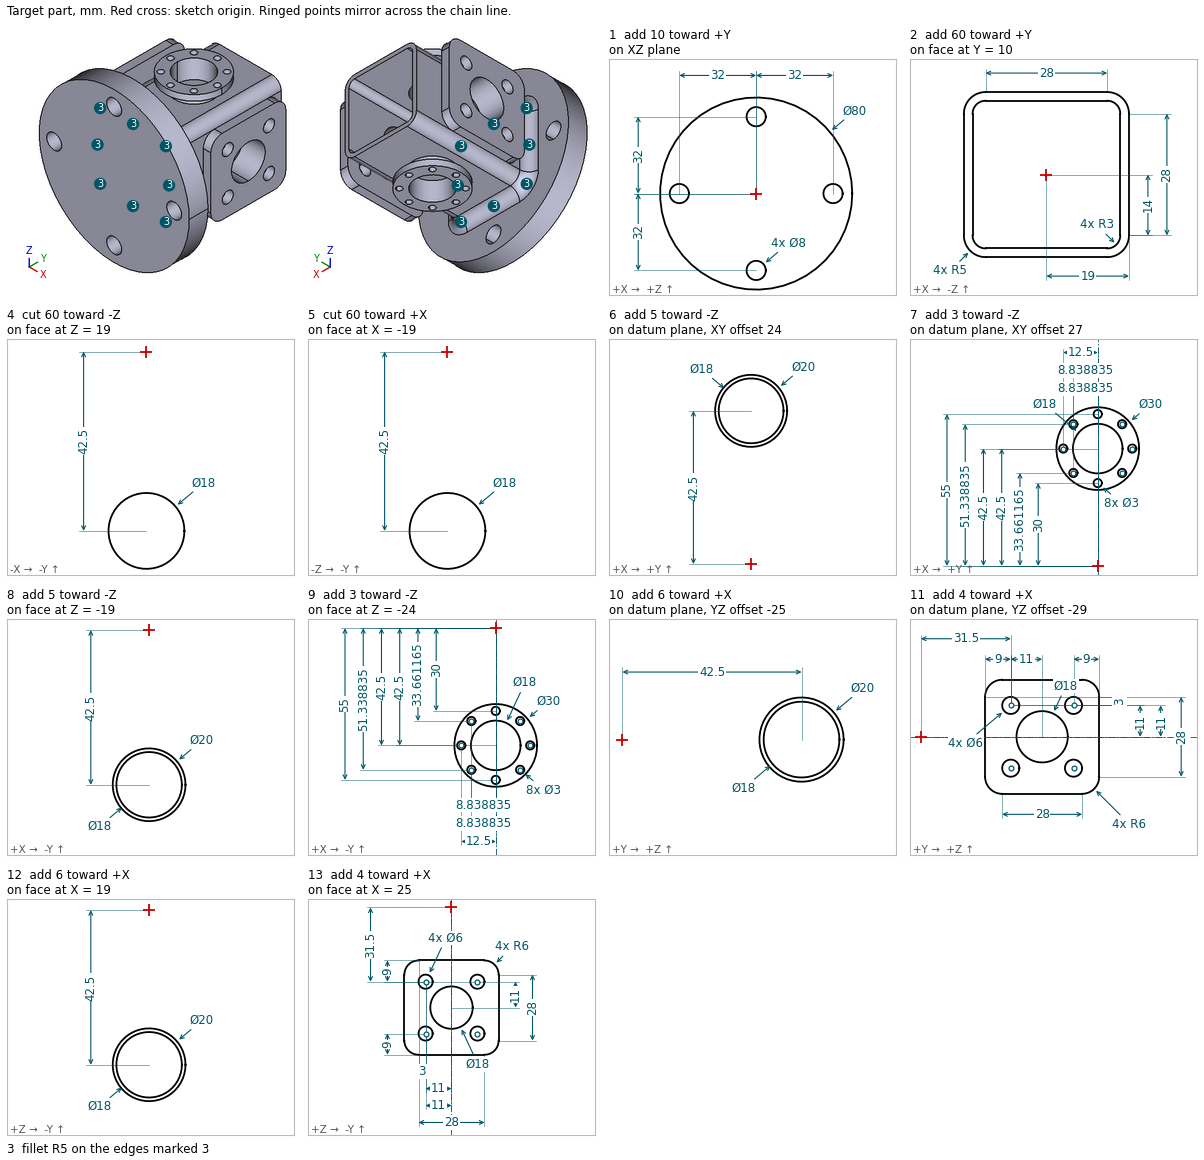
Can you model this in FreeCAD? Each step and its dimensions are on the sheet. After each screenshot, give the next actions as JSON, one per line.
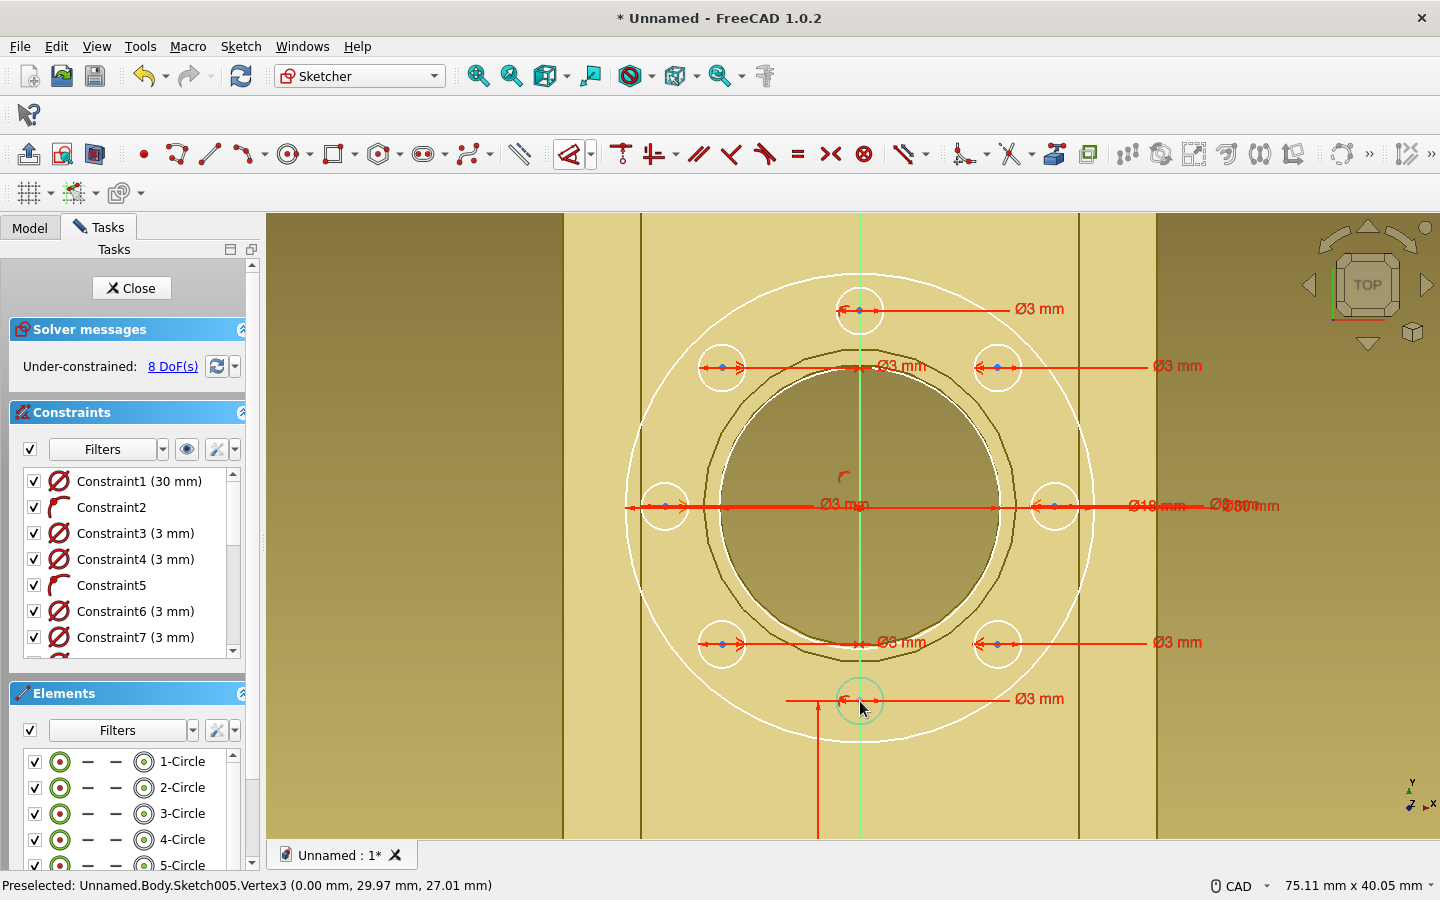
{"action": "left_click", "coordinate": [860, 311]}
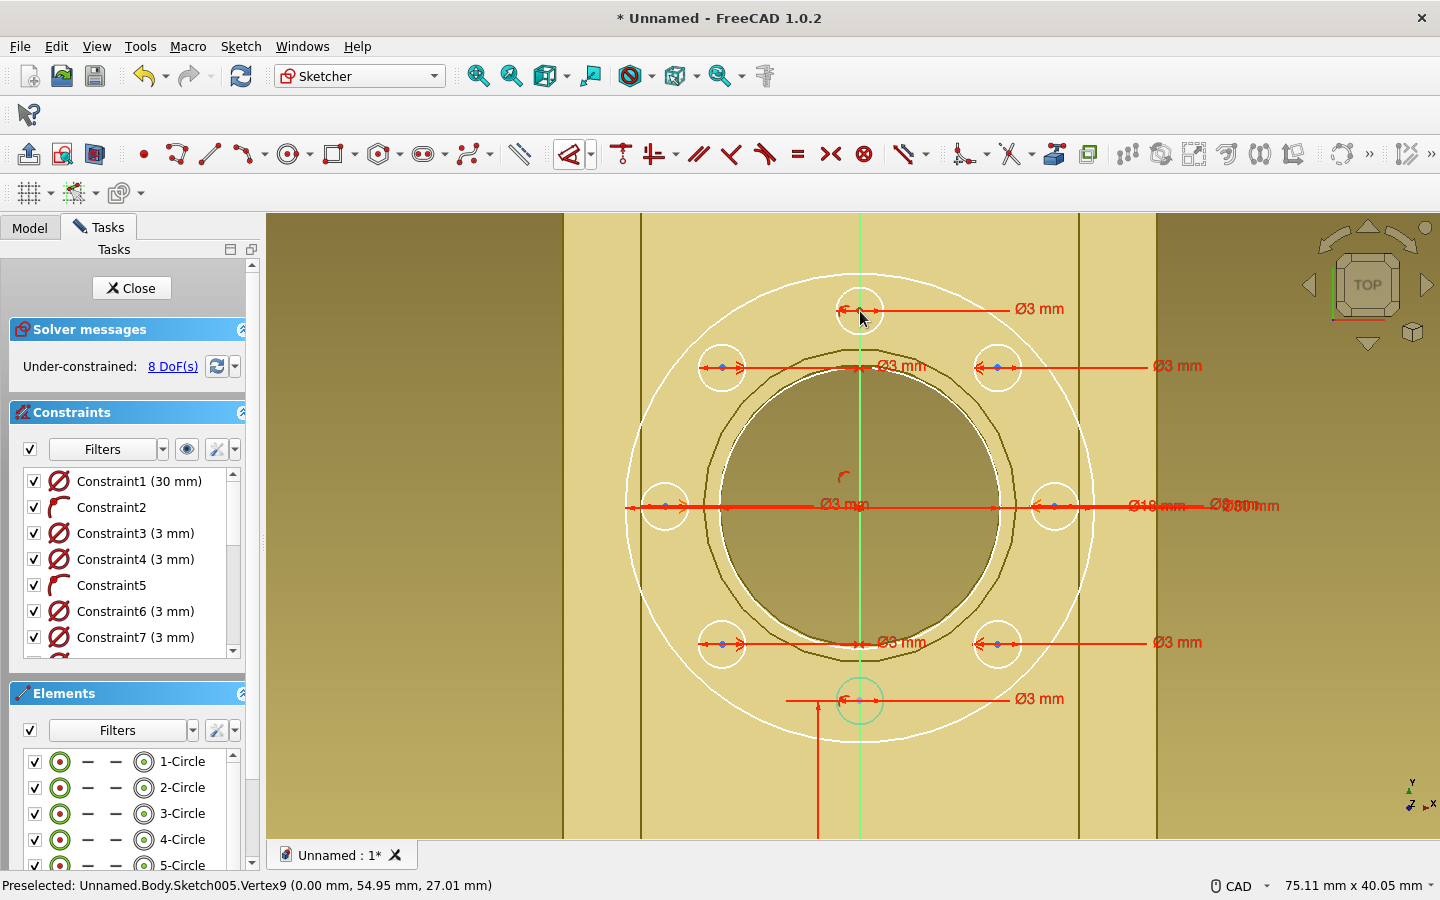
{"action": "key", "text": "i"}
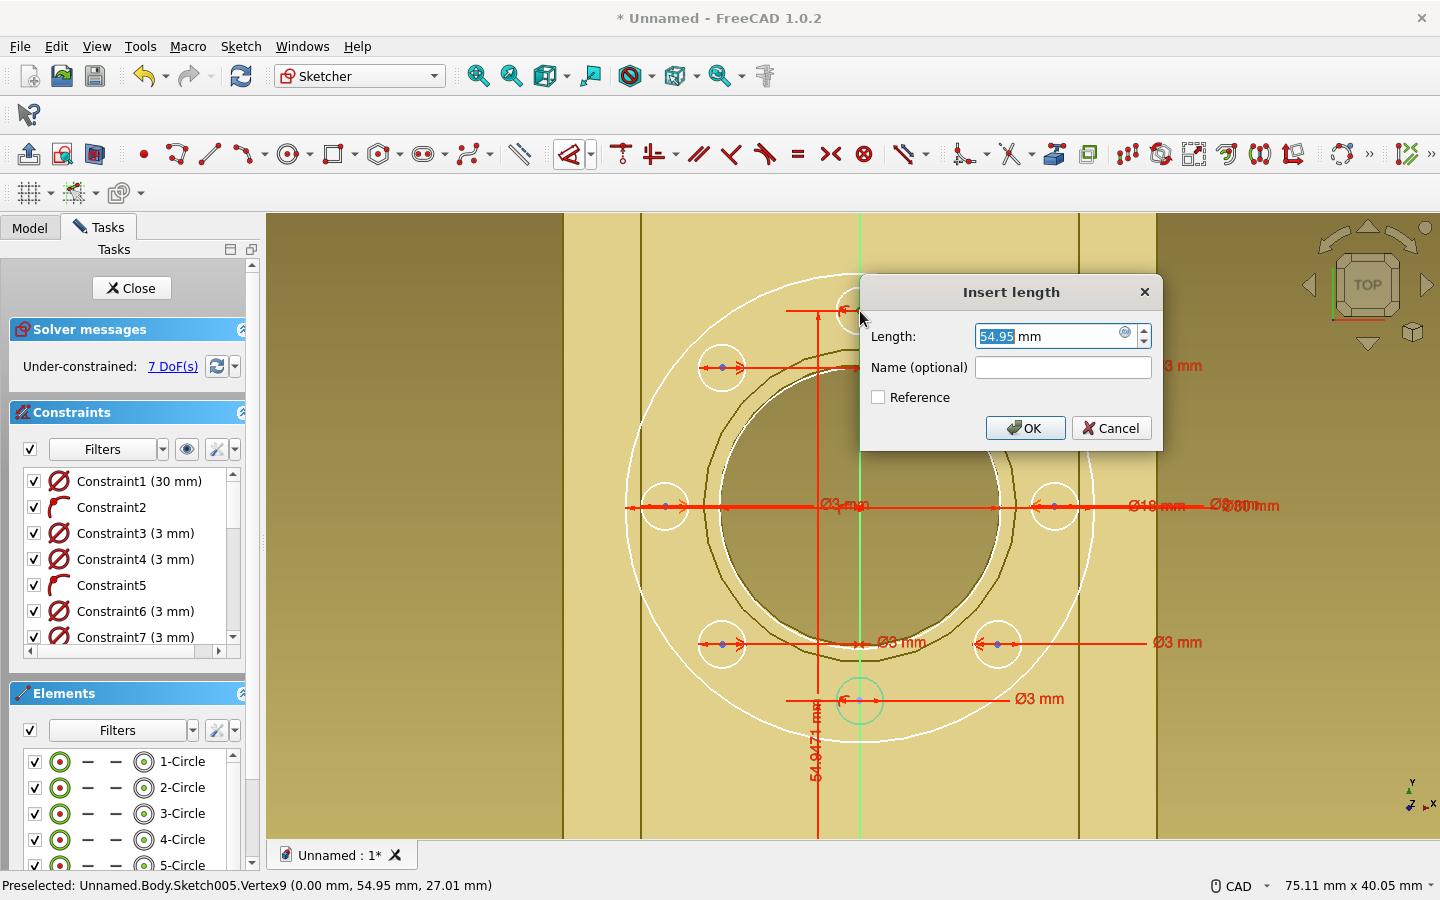
{"action": "type", "text": "55"}
{"action": "key", "text": "Return"}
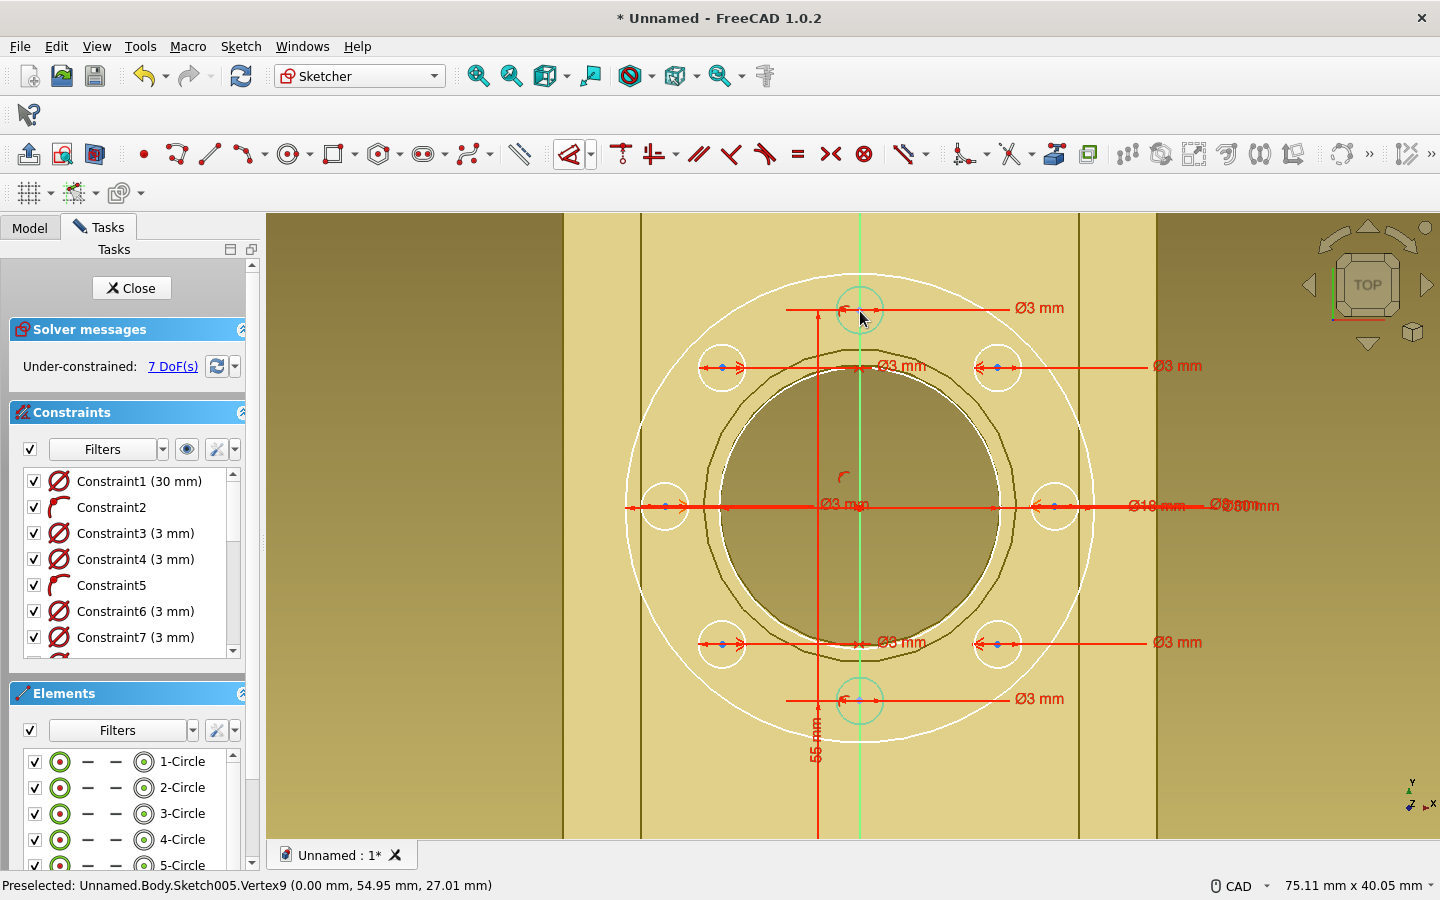
{"action": "left_click", "coordinate": [860, 508]}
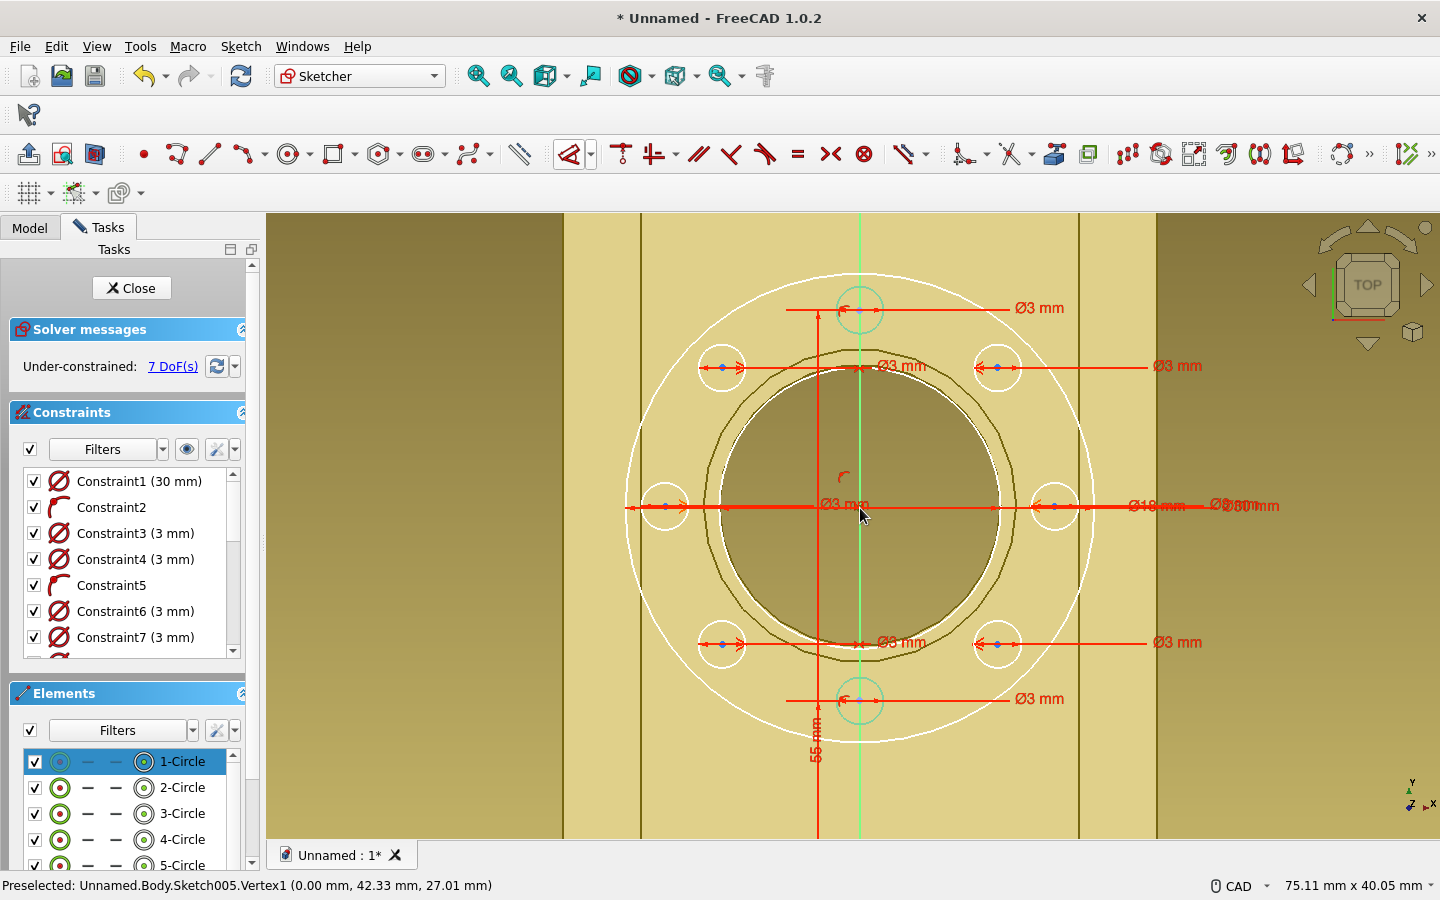
{"action": "left_click", "coordinate": [590, 154]}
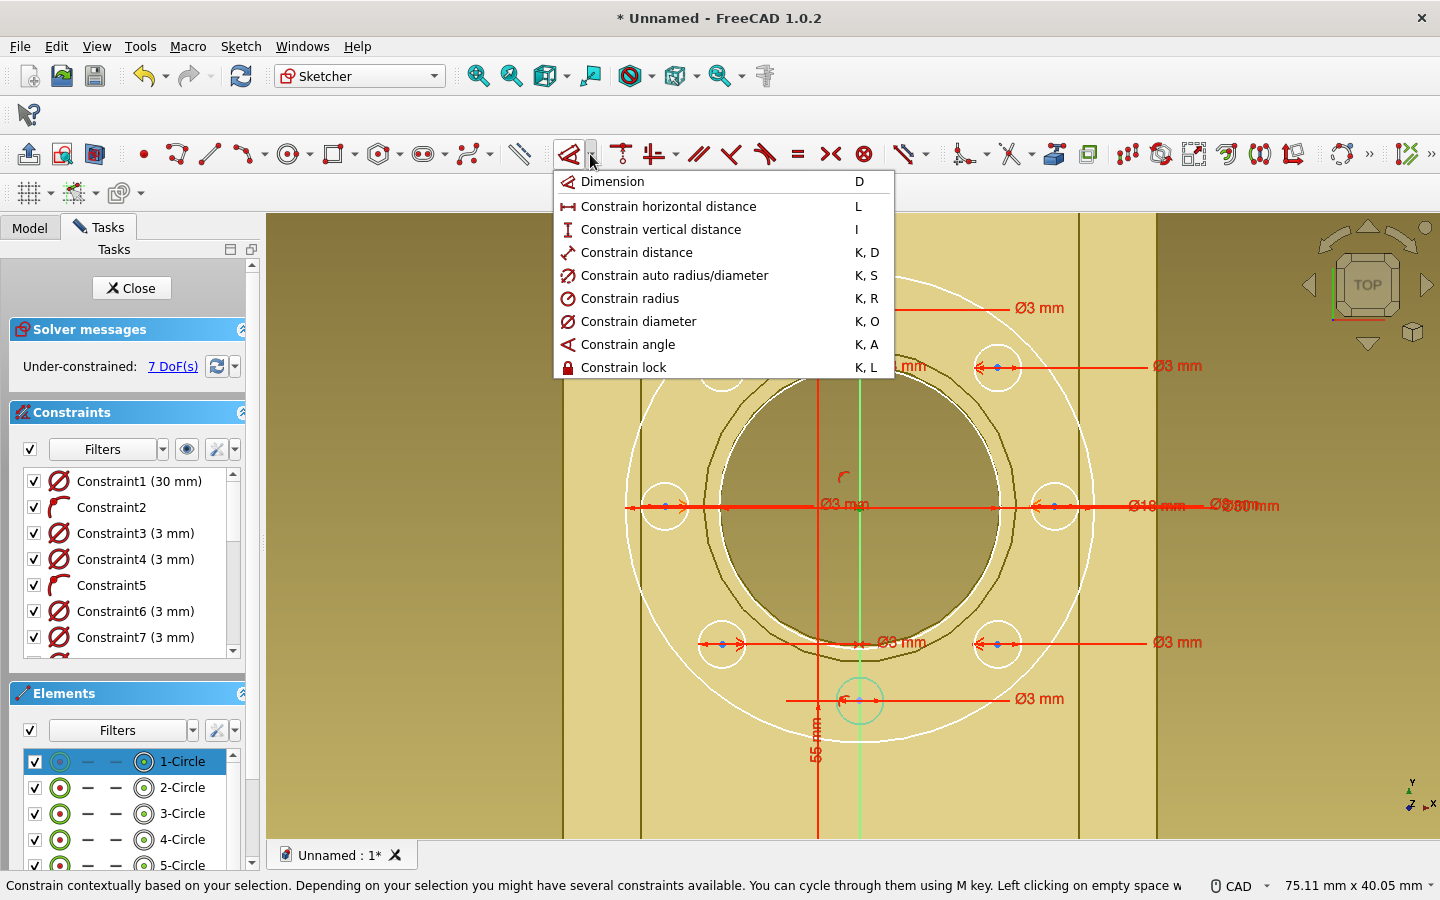
{"action": "left_click", "coordinate": [724, 230]}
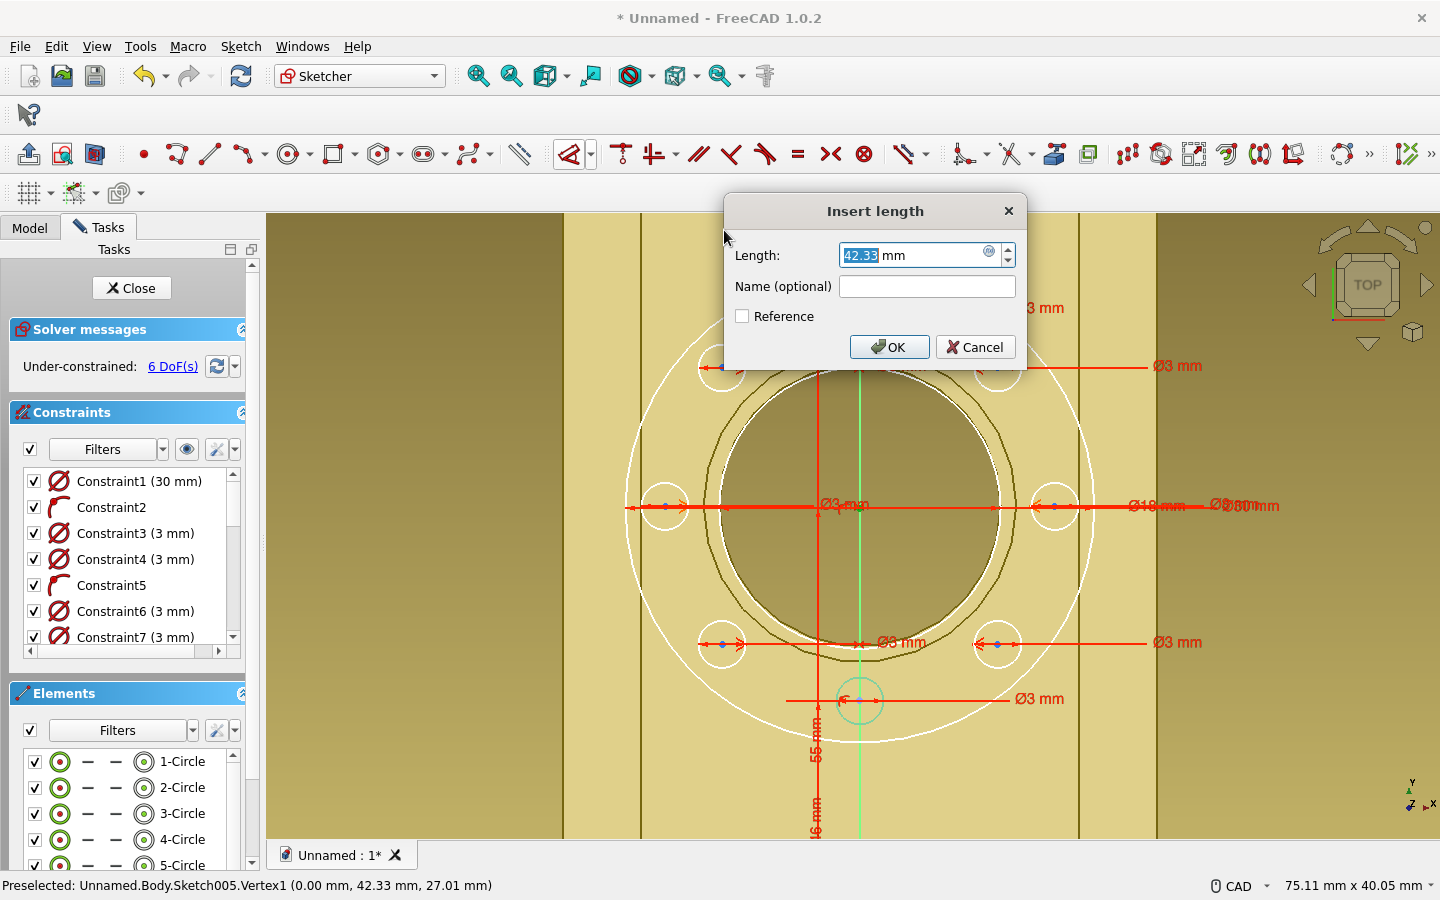
{"action": "type", "text": "42.5"}
{"action": "key", "text": "Return"}